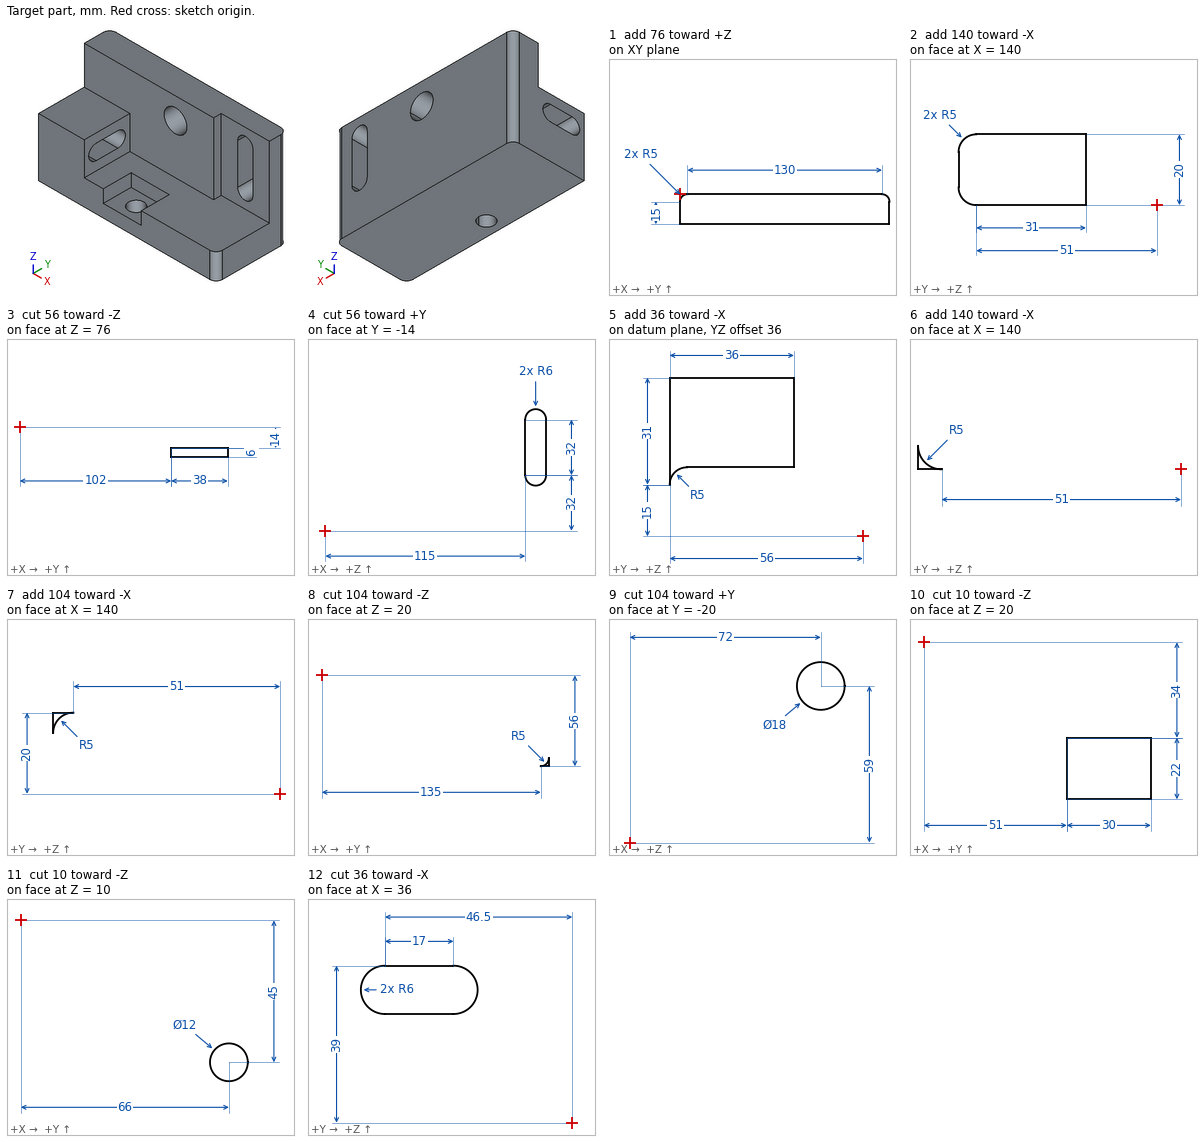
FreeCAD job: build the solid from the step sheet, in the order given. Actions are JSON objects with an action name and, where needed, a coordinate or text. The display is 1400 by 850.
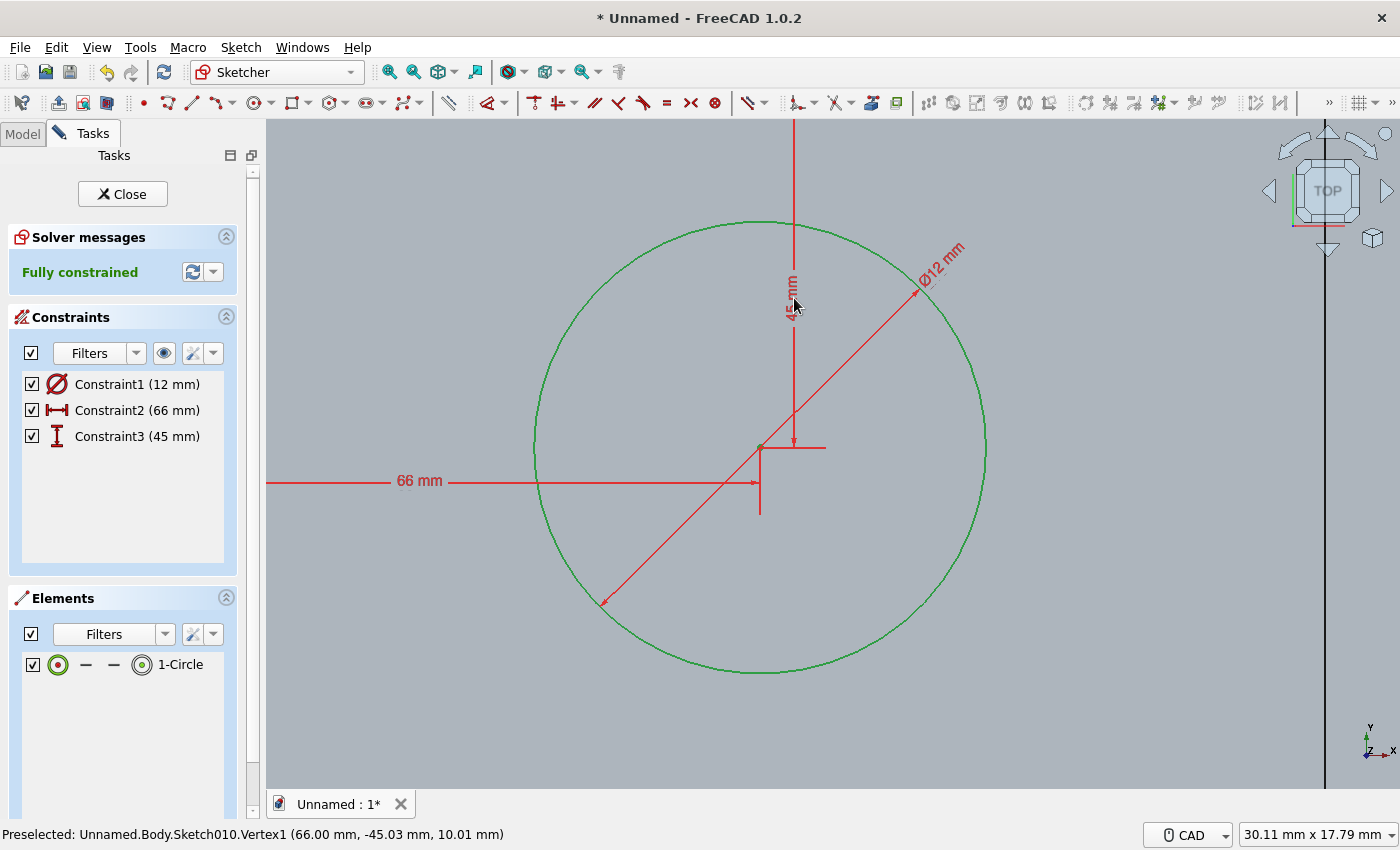
{"action": "left_click", "coordinate": [123, 194]}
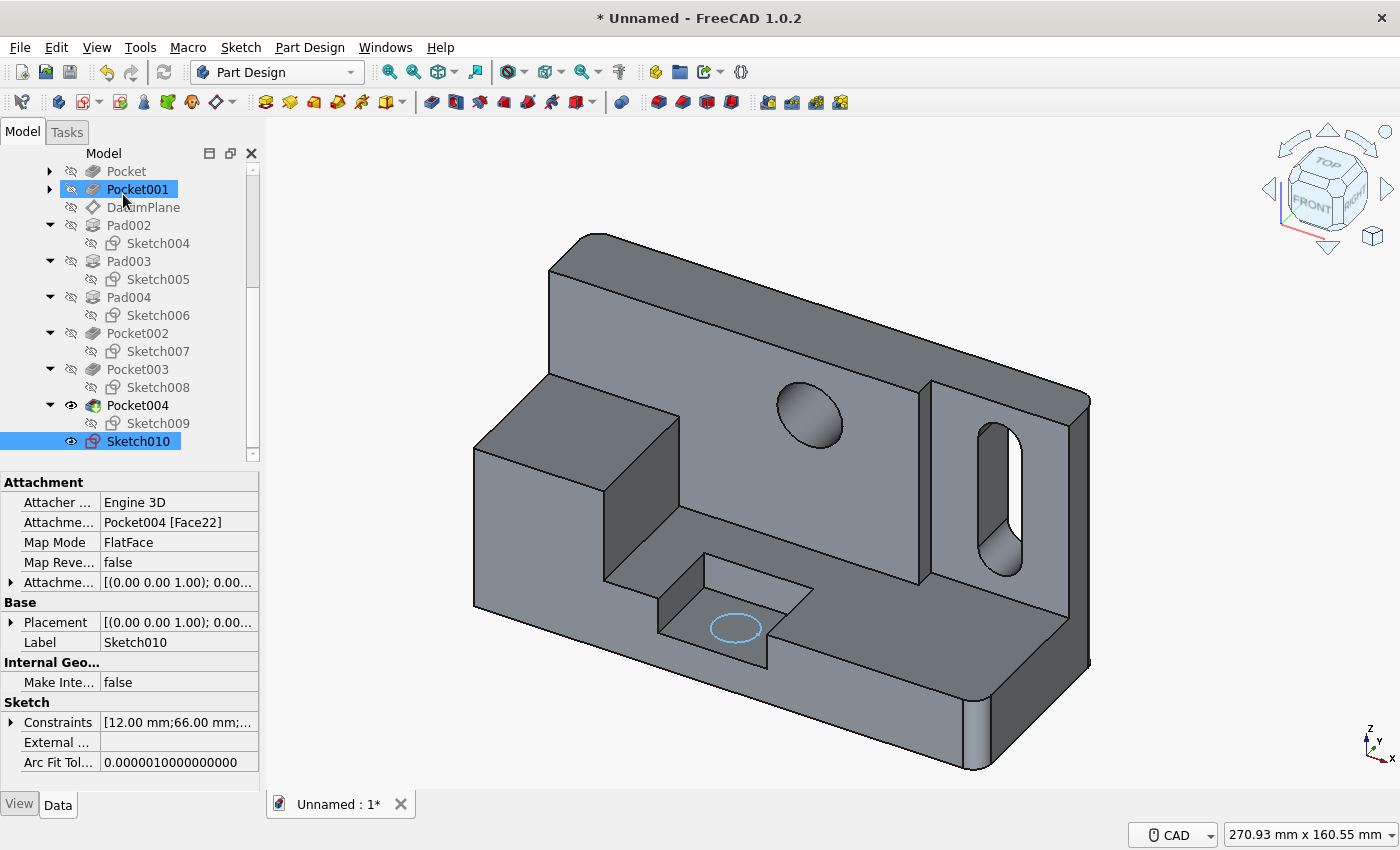
{"action": "left_click", "coordinate": [432, 102]}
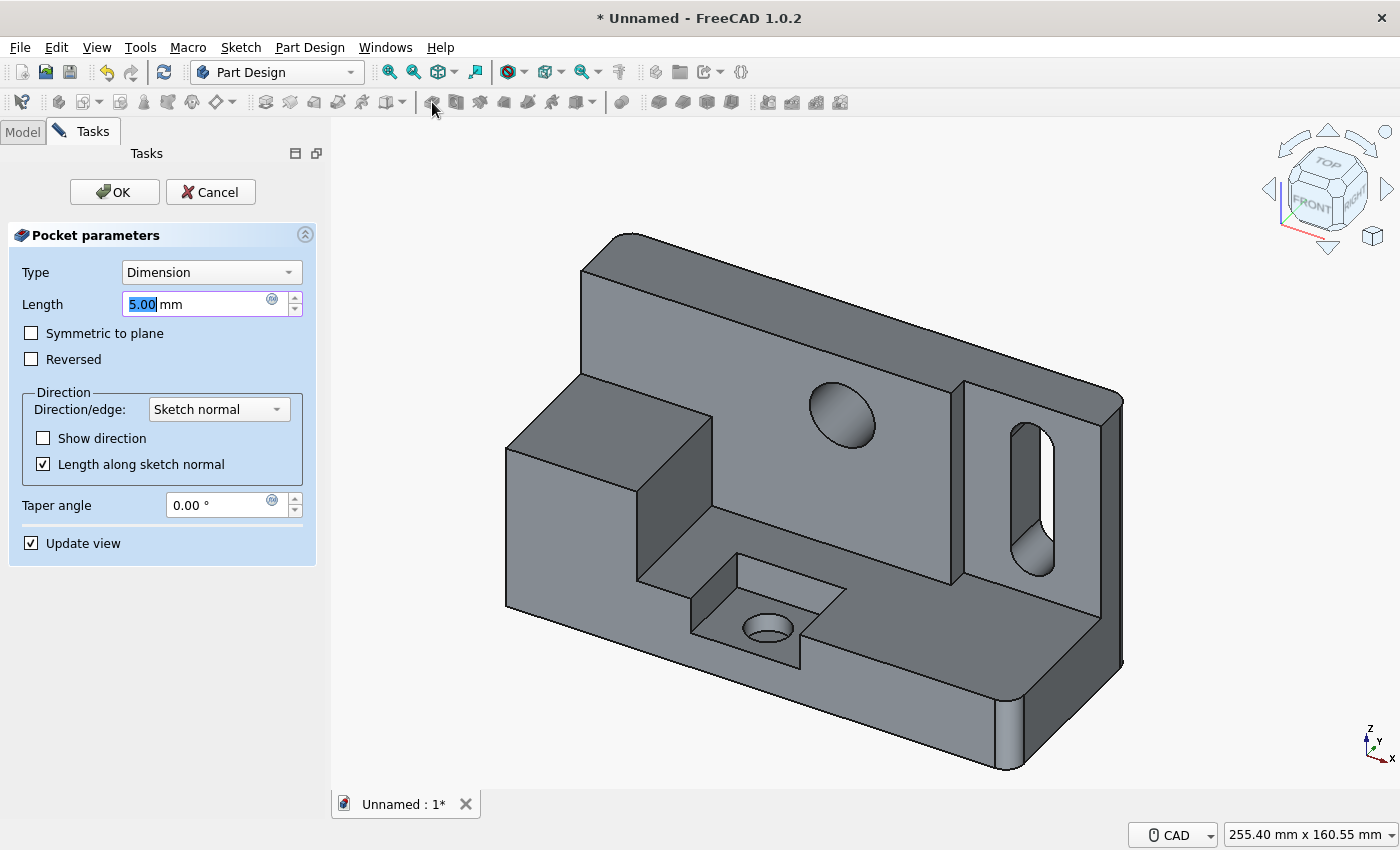
{"action": "type", "text": "10"}
{"action": "key", "text": "Tab"}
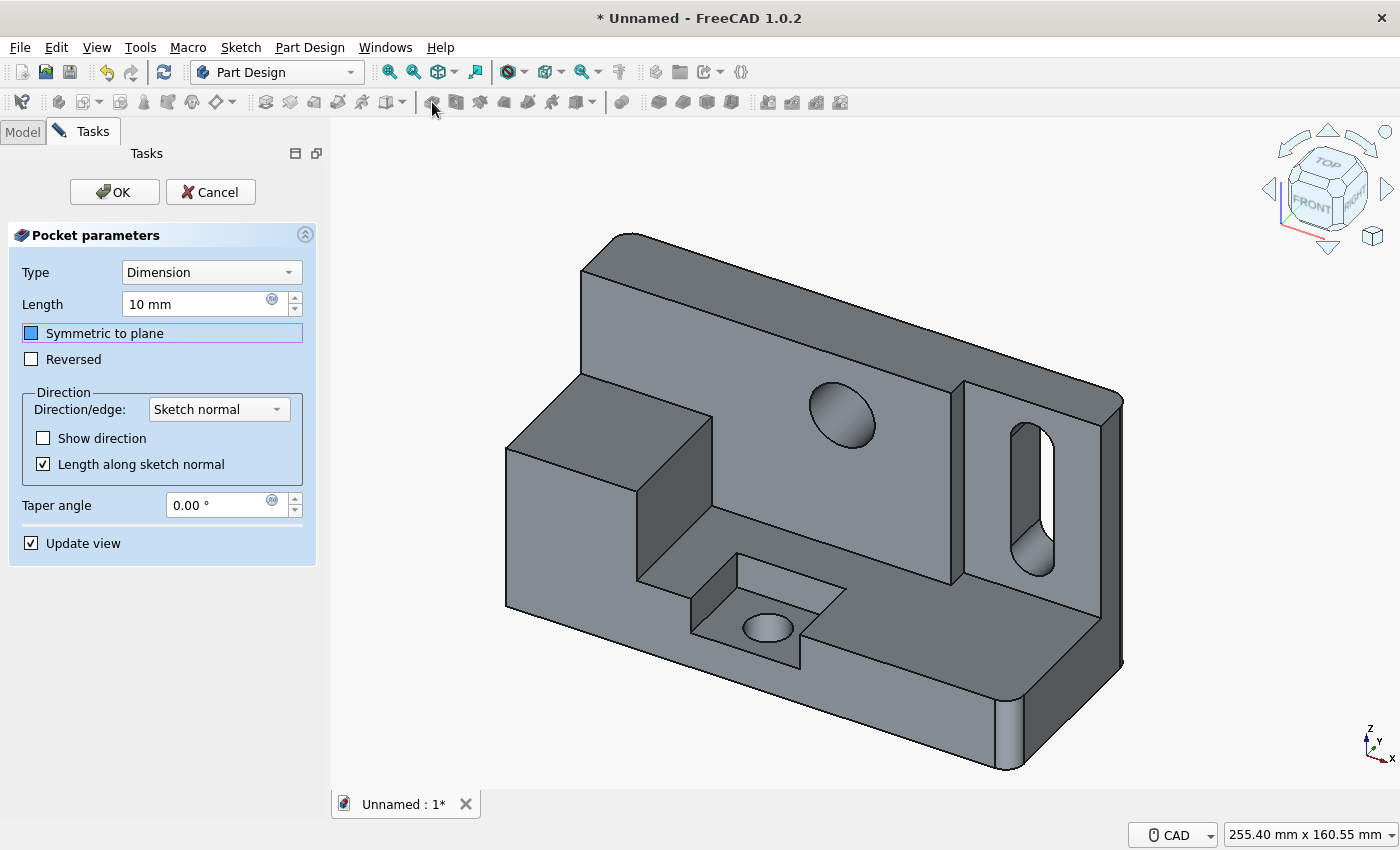
{"action": "left_click", "coordinate": [115, 192]}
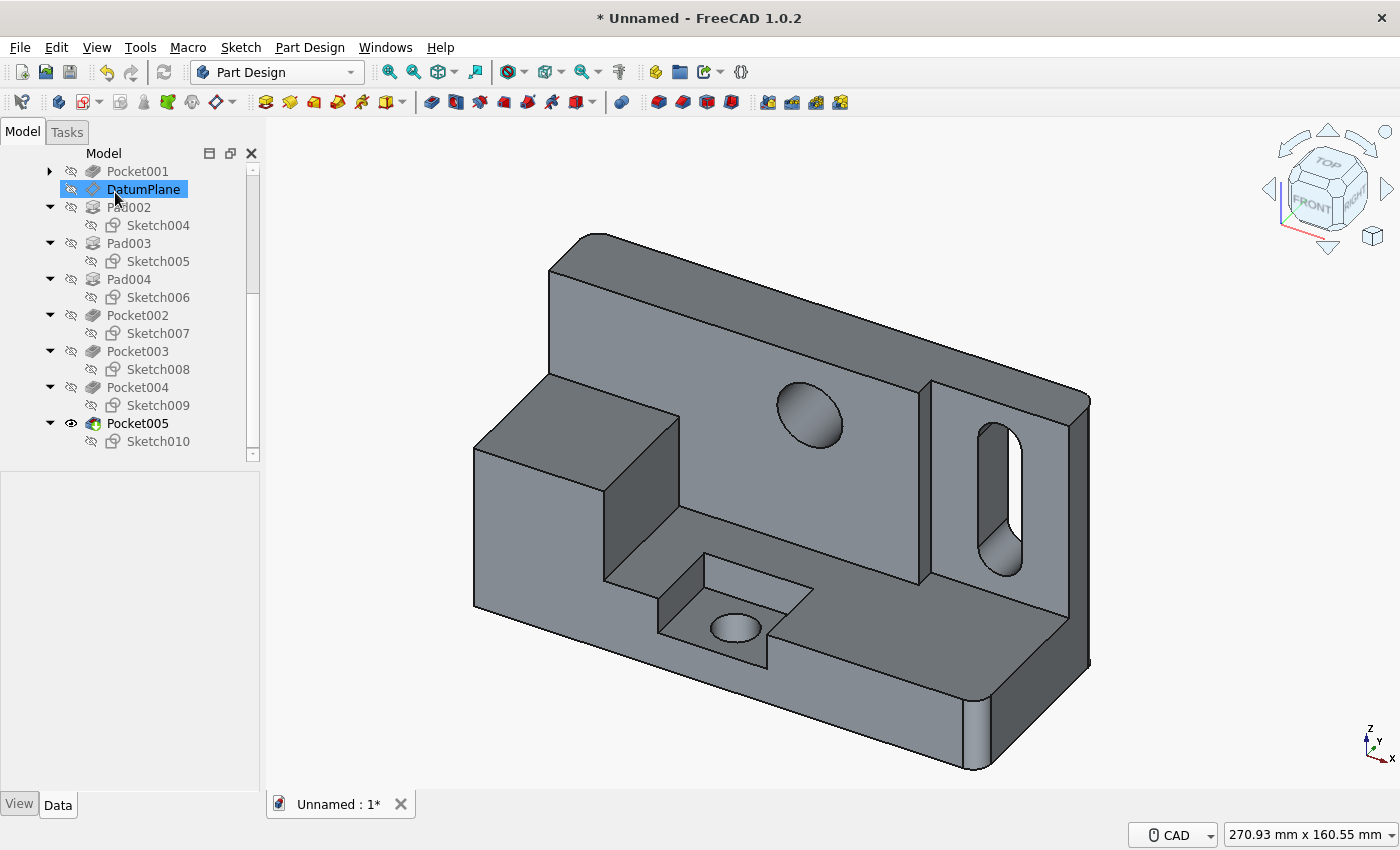
{"action": "left_click", "coordinate": [642, 498]}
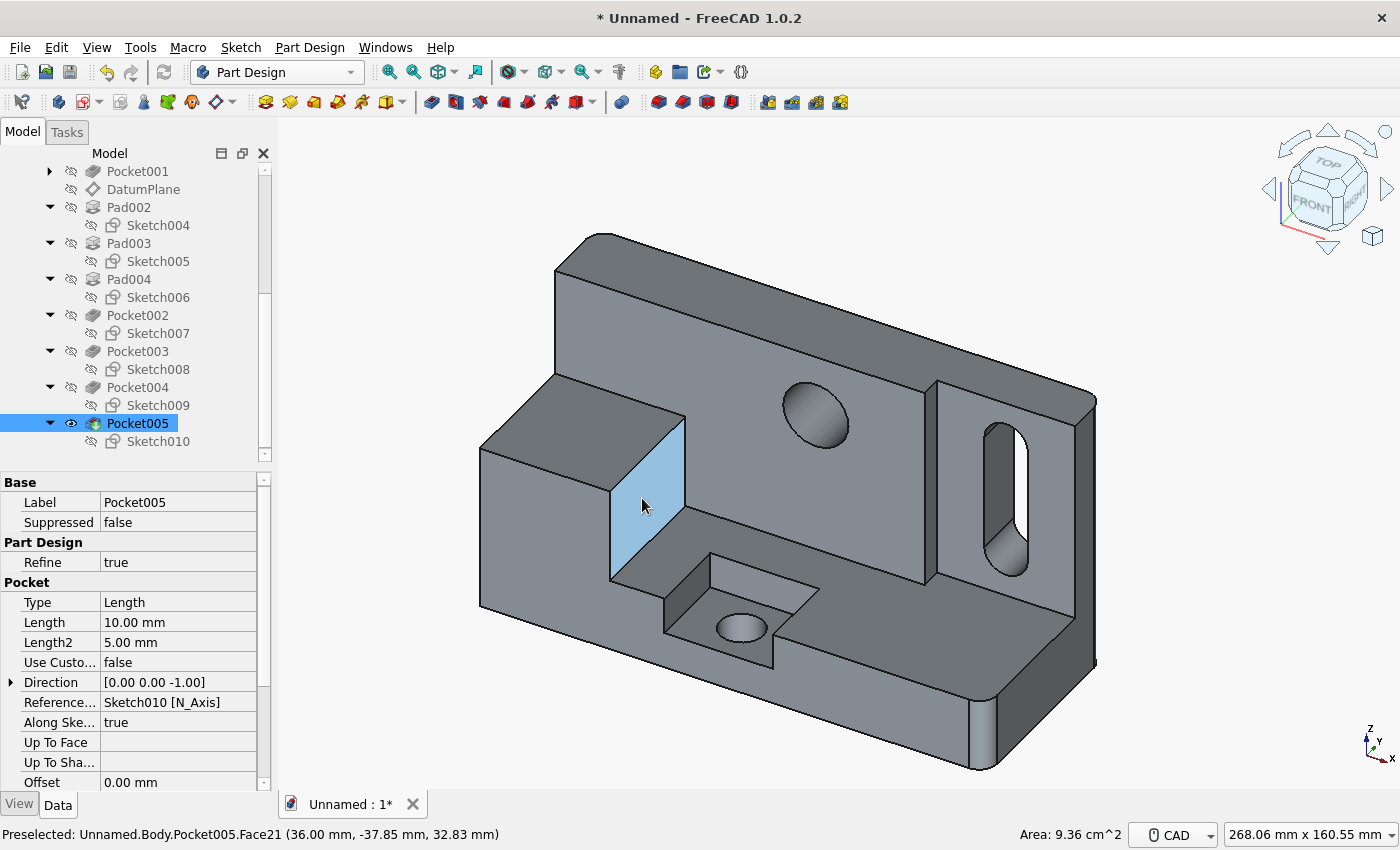
{"action": "left_click", "coordinate": [84, 102]}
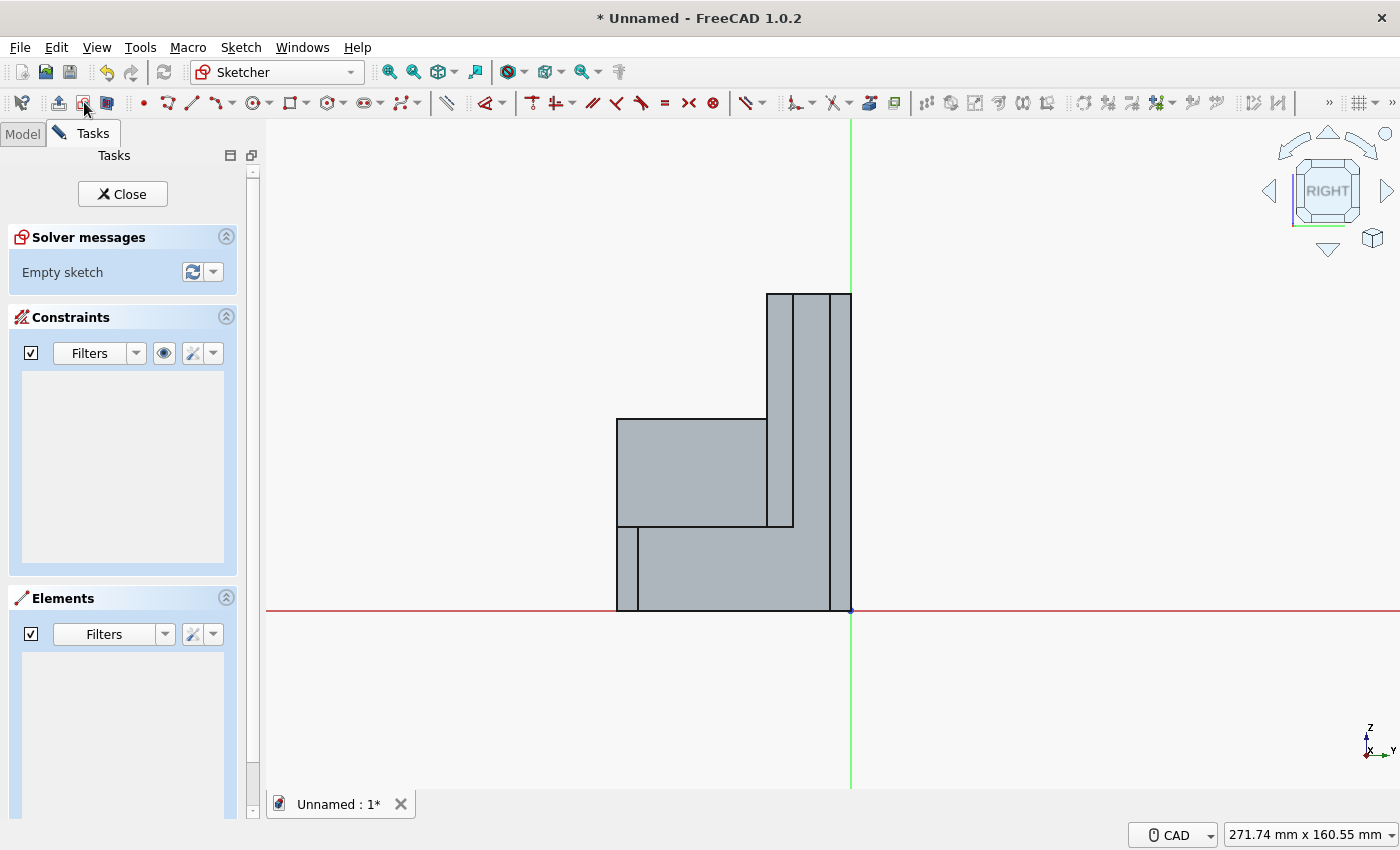
{"action": "key", "text": "q s"}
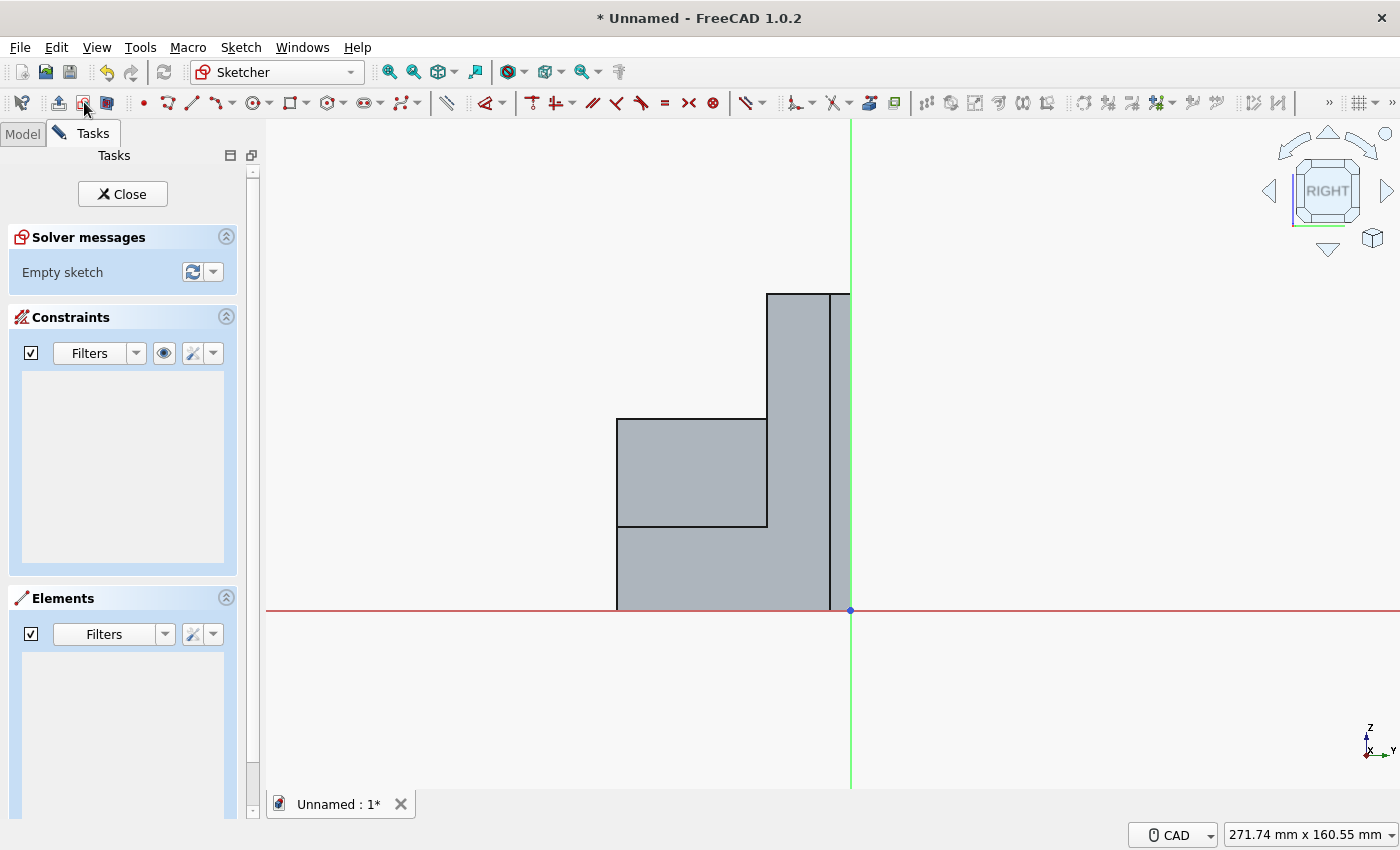
{"action": "scroll", "coordinate": [728, 573], "scroll_direction": "up", "scroll_amount": 5}